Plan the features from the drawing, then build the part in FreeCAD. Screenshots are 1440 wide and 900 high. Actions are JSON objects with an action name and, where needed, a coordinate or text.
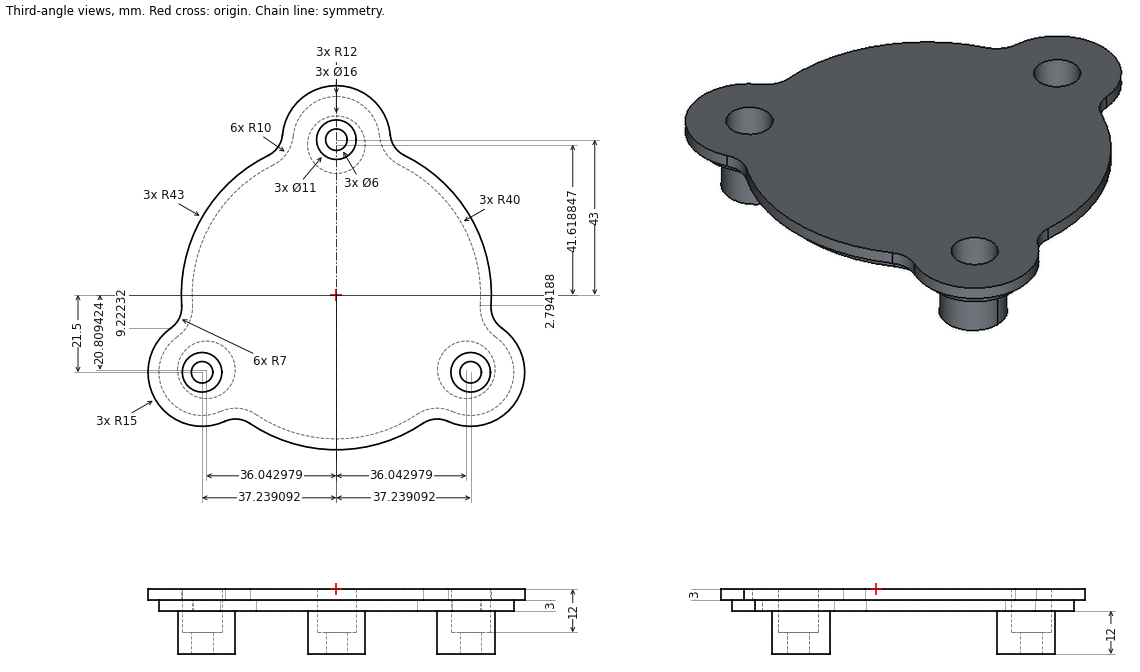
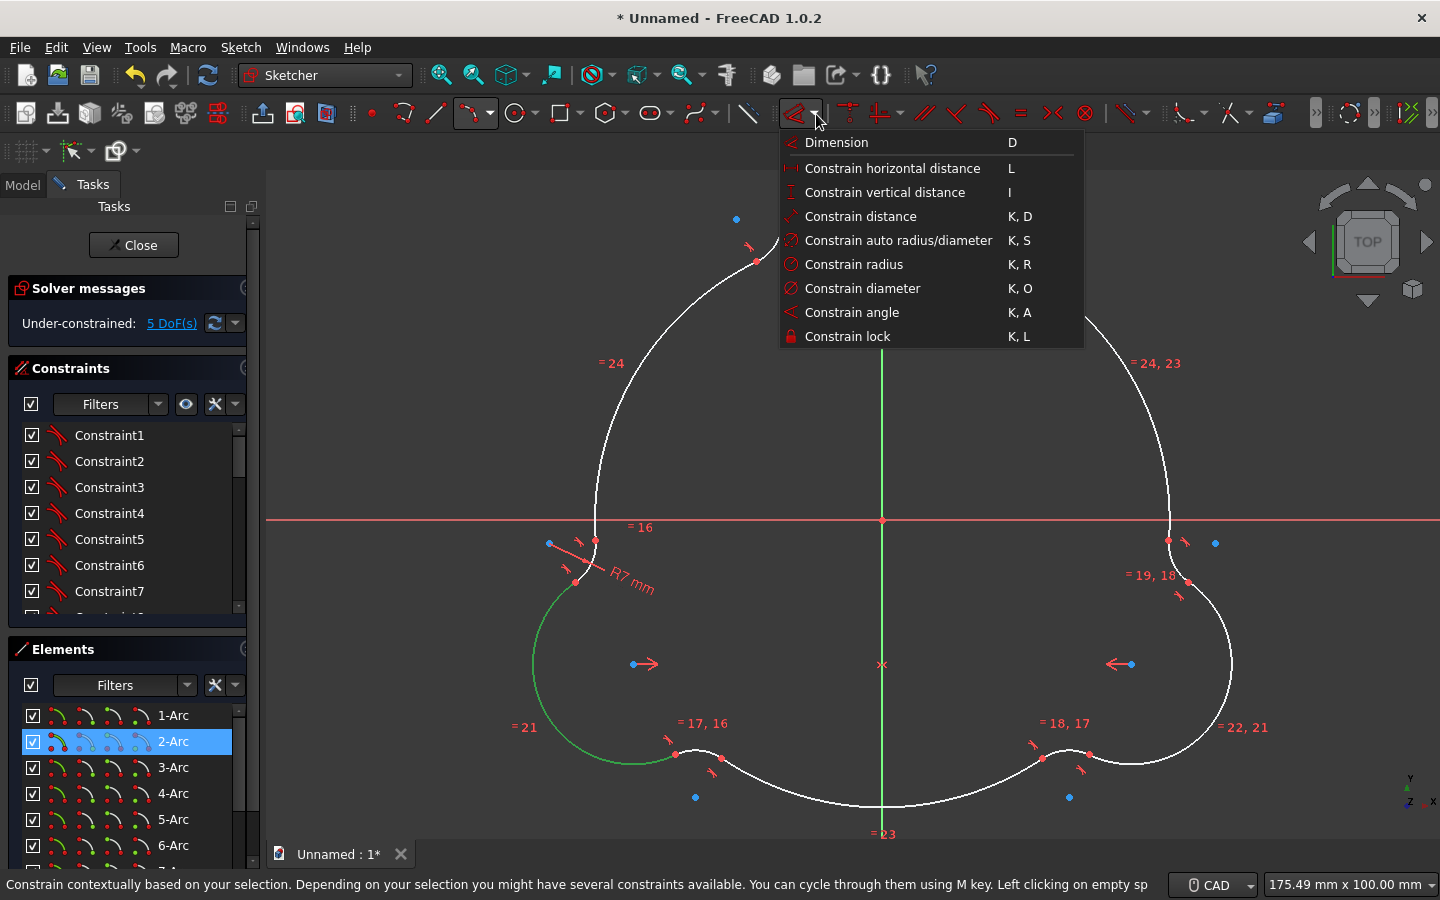
{"action": "left_click", "coordinate": [932, 264]}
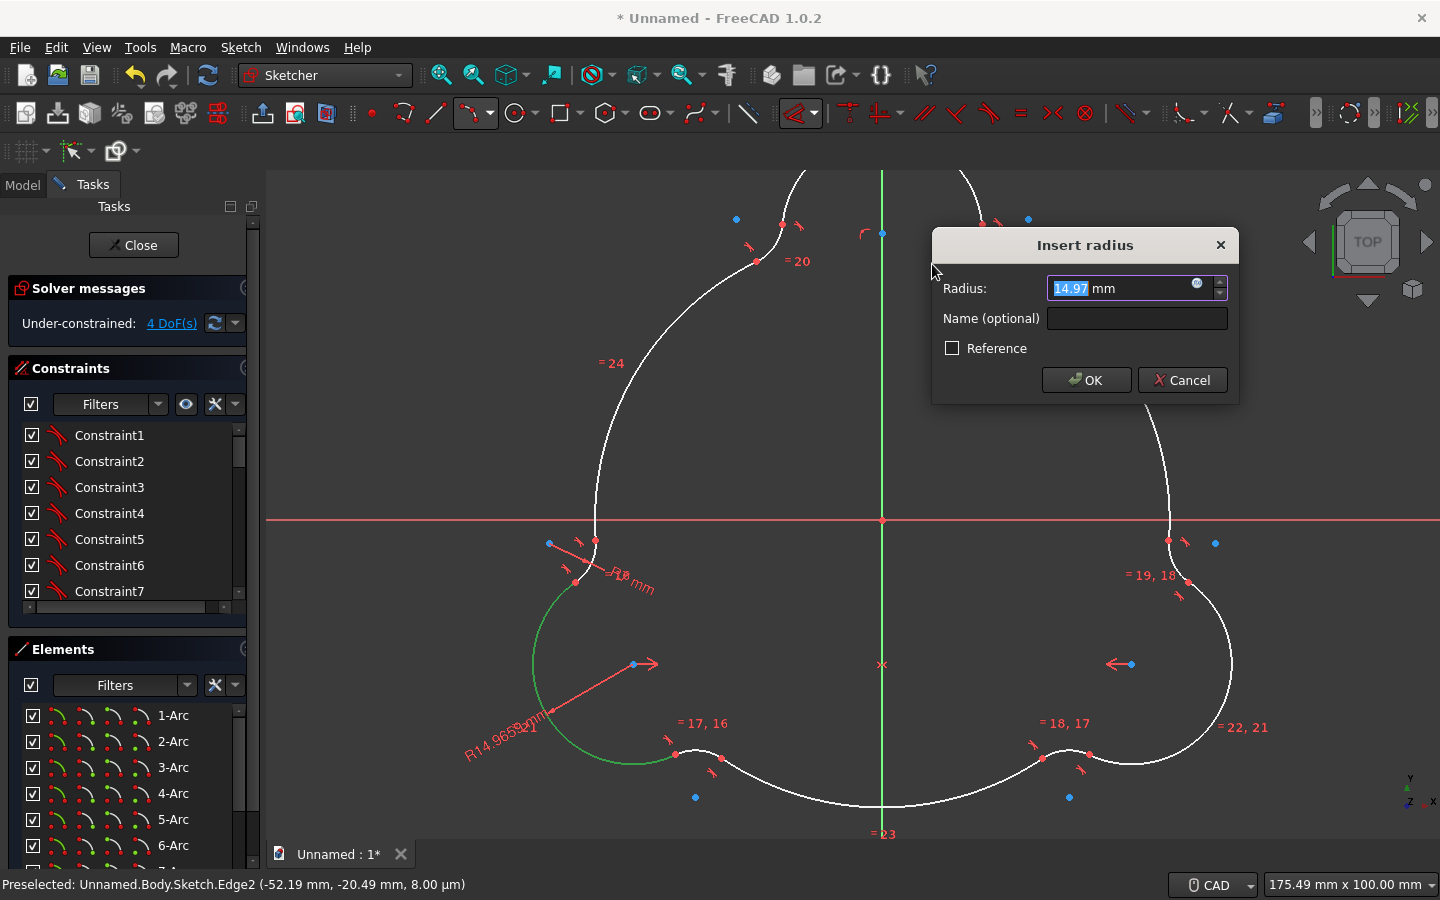
{"action": "type", "text": "15"}
{"action": "key", "text": "Return"}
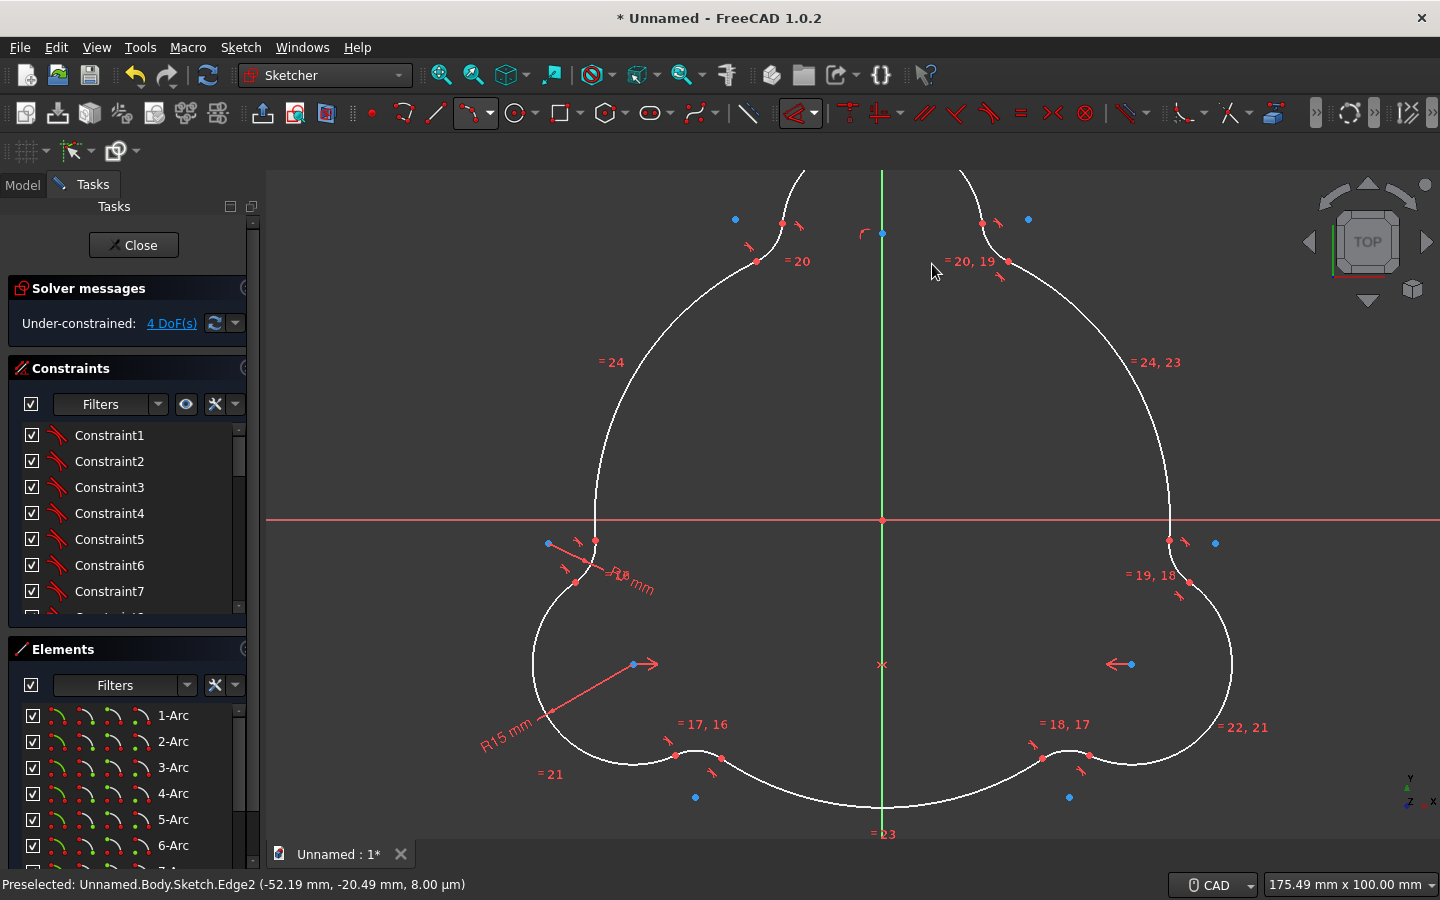
{"action": "left_click", "coordinate": [815, 800]}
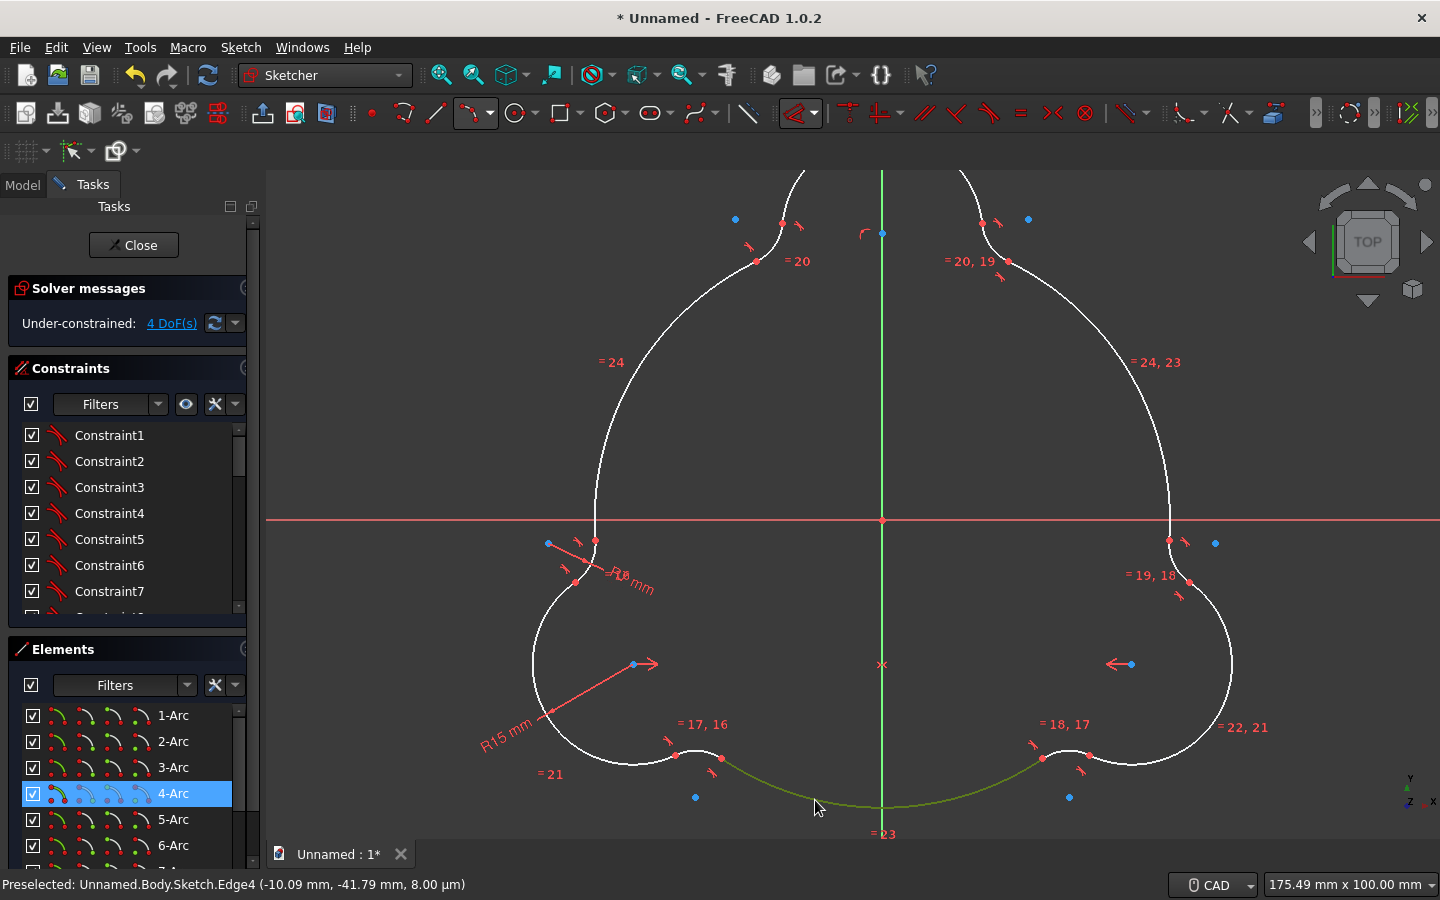
{"action": "left_click", "coordinate": [816, 114]}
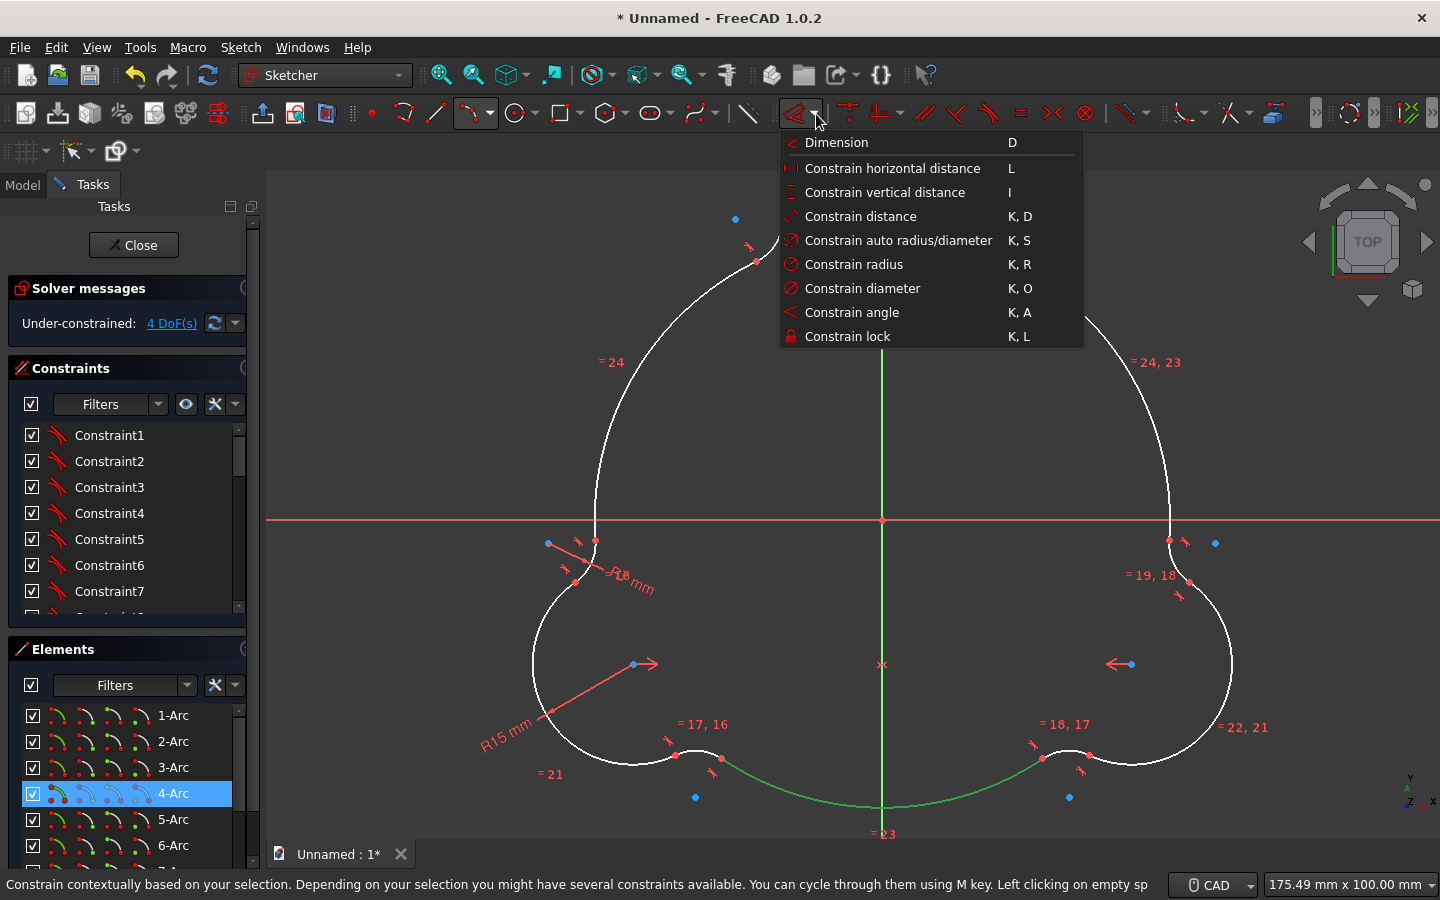
{"action": "left_click", "coordinate": [932, 264]}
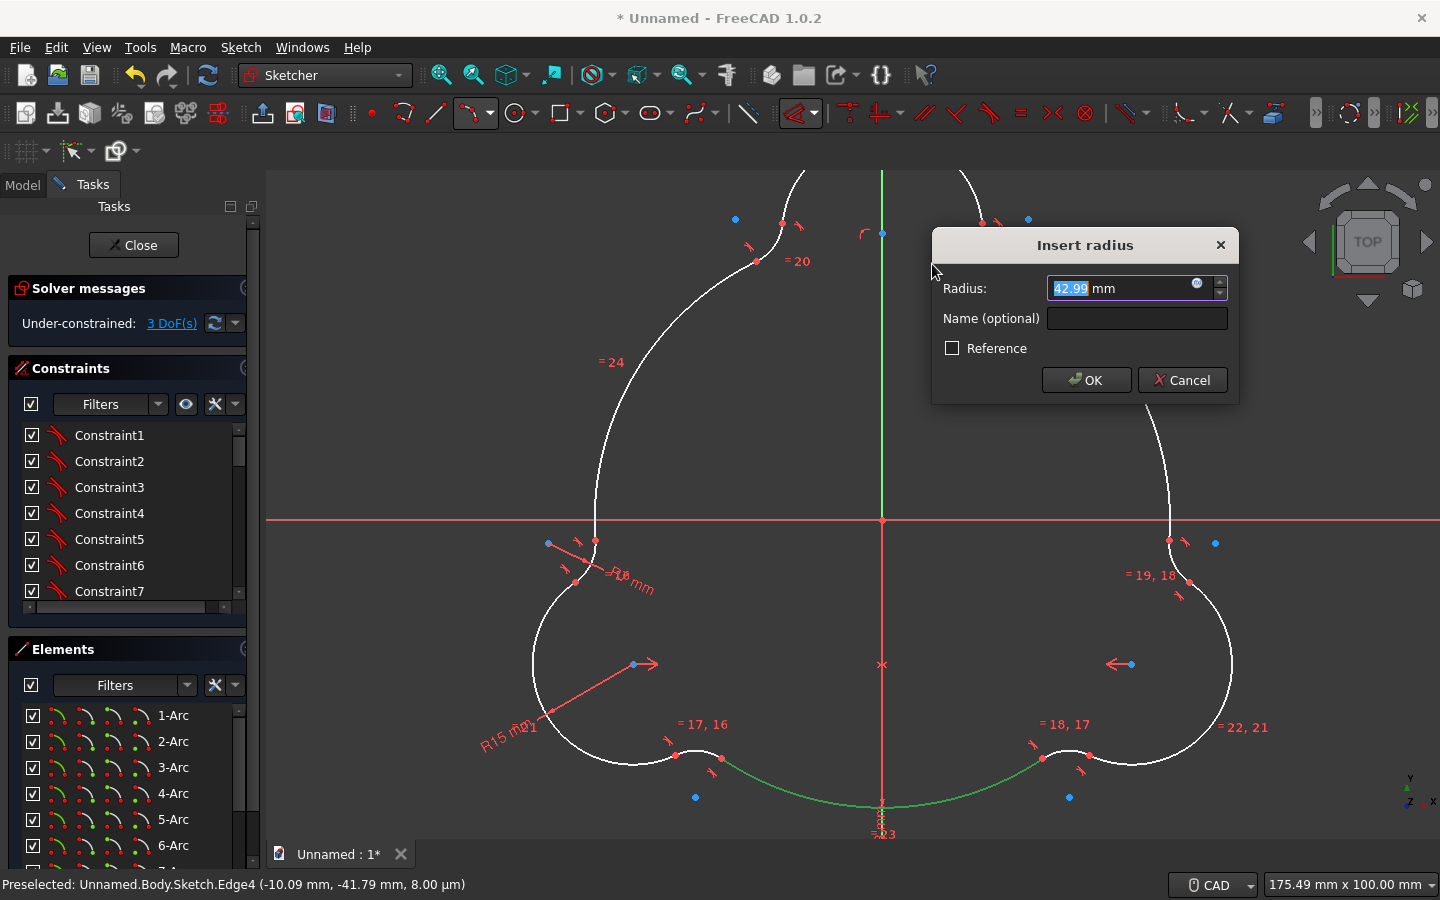
{"action": "type", "text": "43"}
{"action": "key", "text": "Return"}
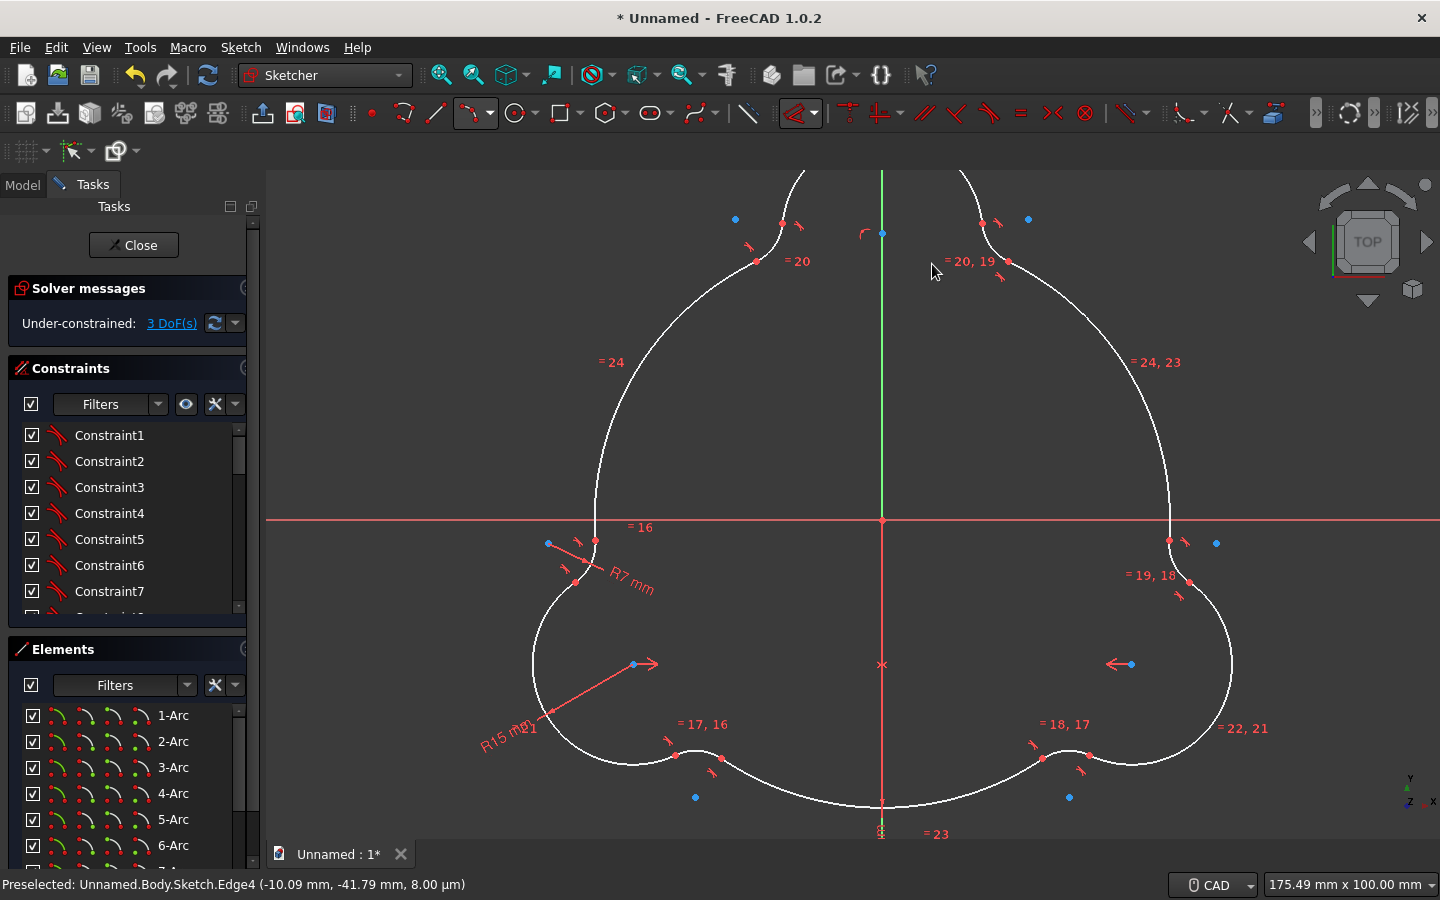
{"action": "left_click", "coordinate": [882, 234]}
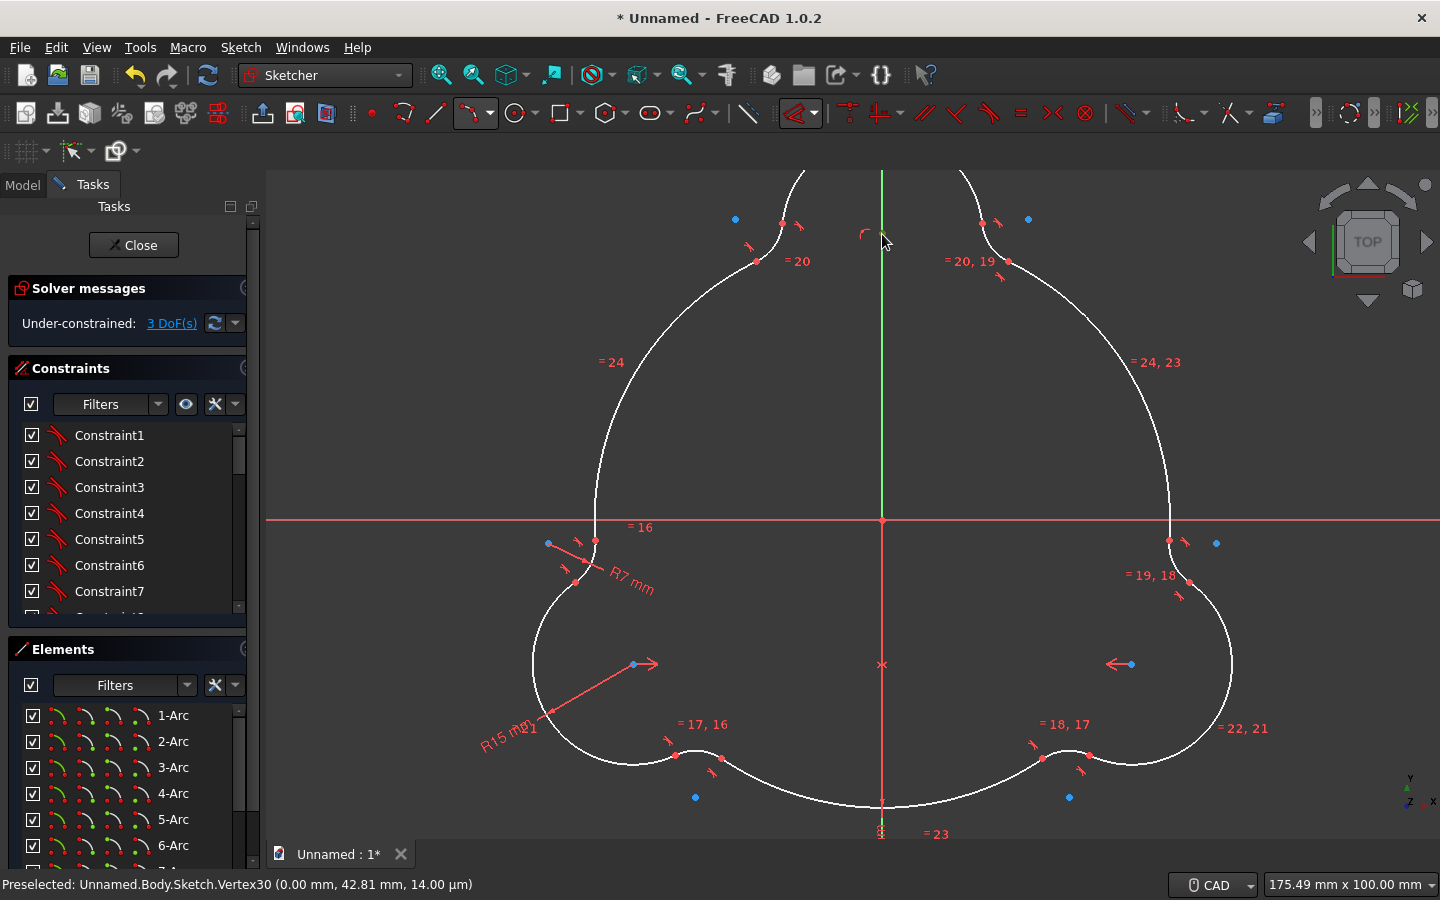
{"action": "key", "text": "i"}